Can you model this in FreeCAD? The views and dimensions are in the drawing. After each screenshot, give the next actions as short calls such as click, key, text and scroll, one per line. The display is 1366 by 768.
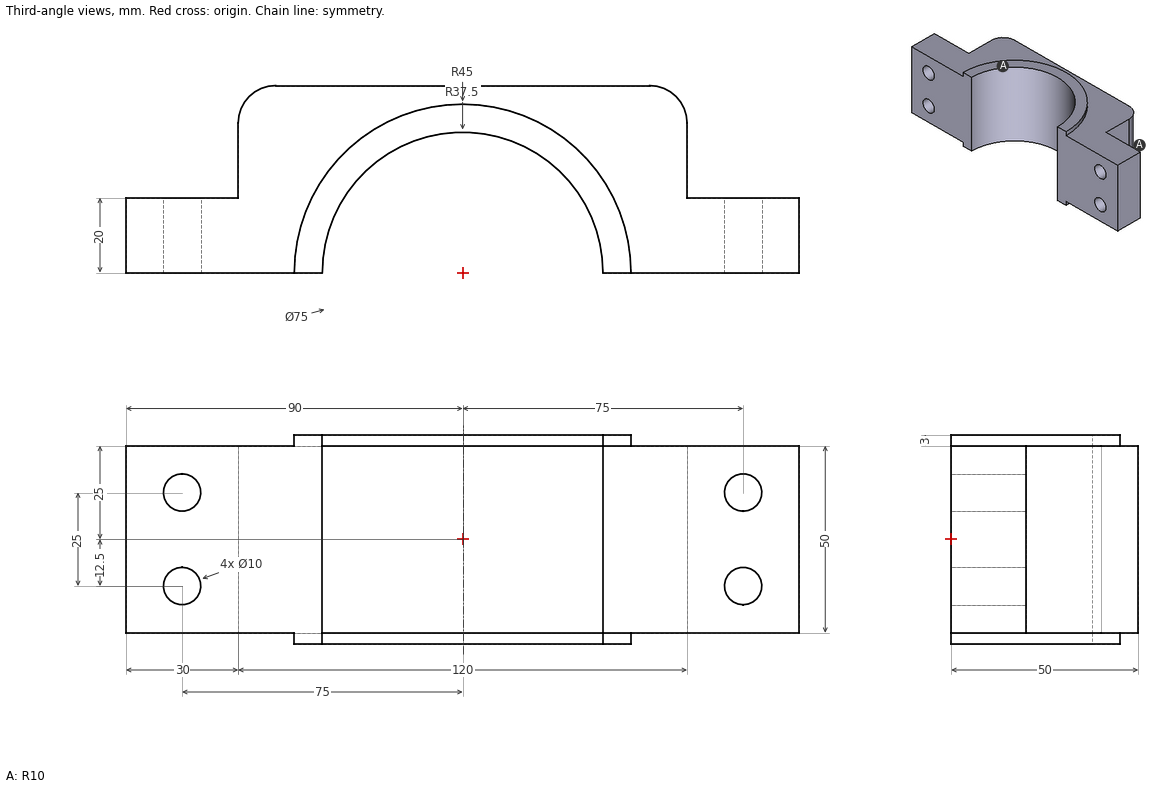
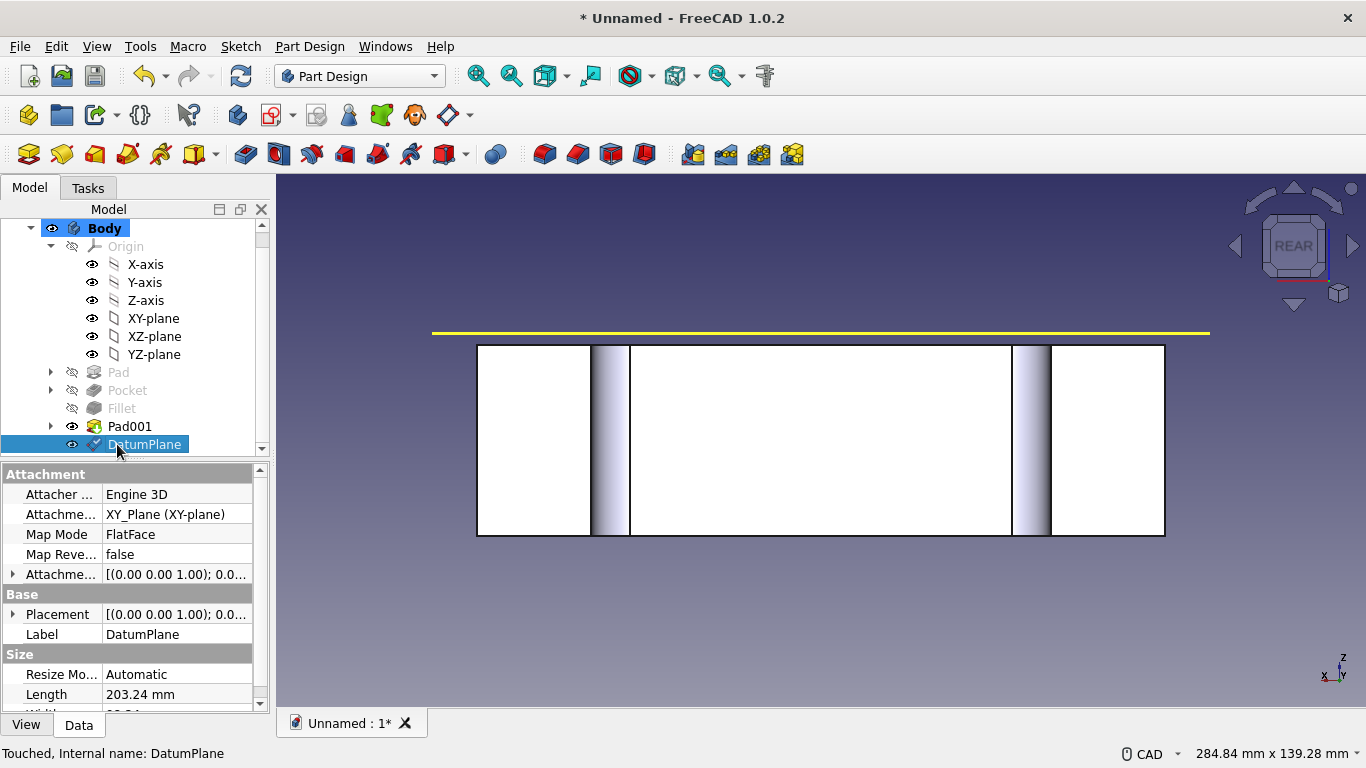
click(270, 116)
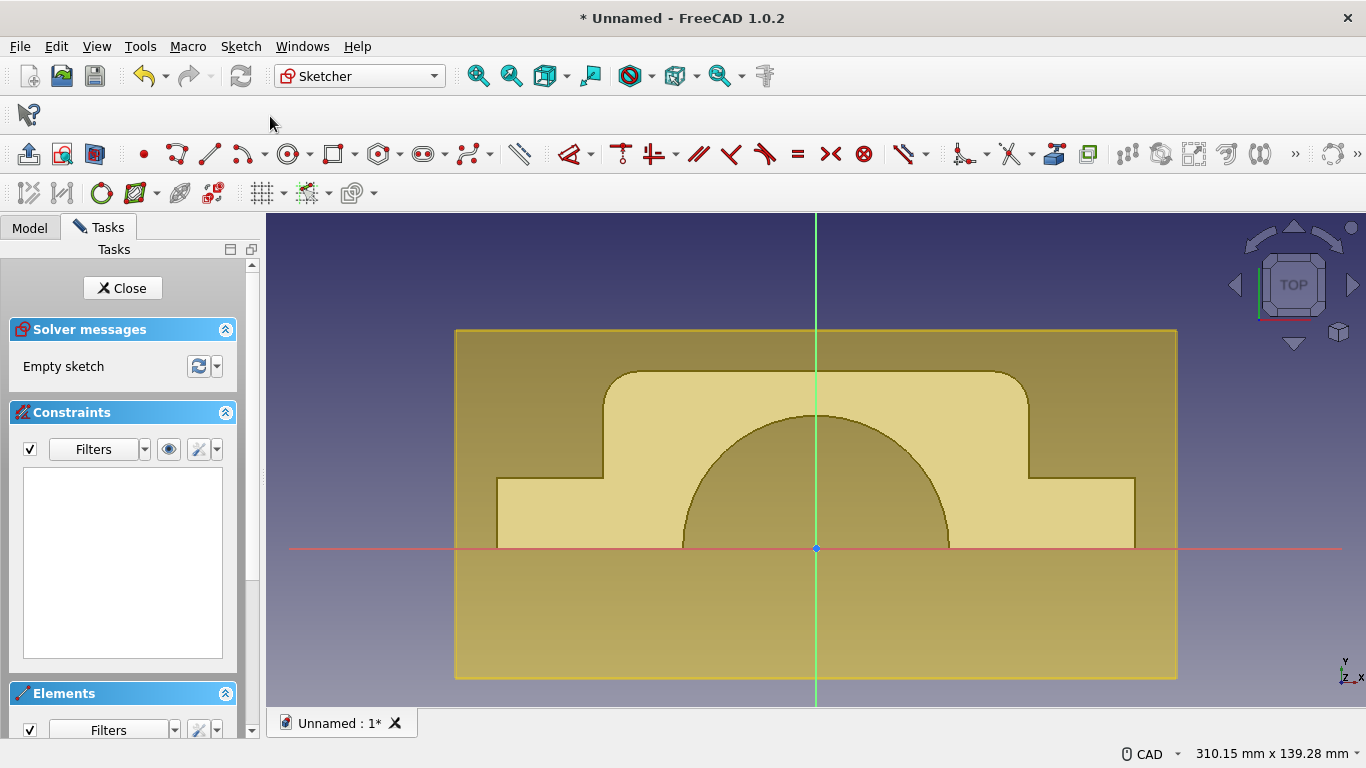
scroll(899, 480, up, 3)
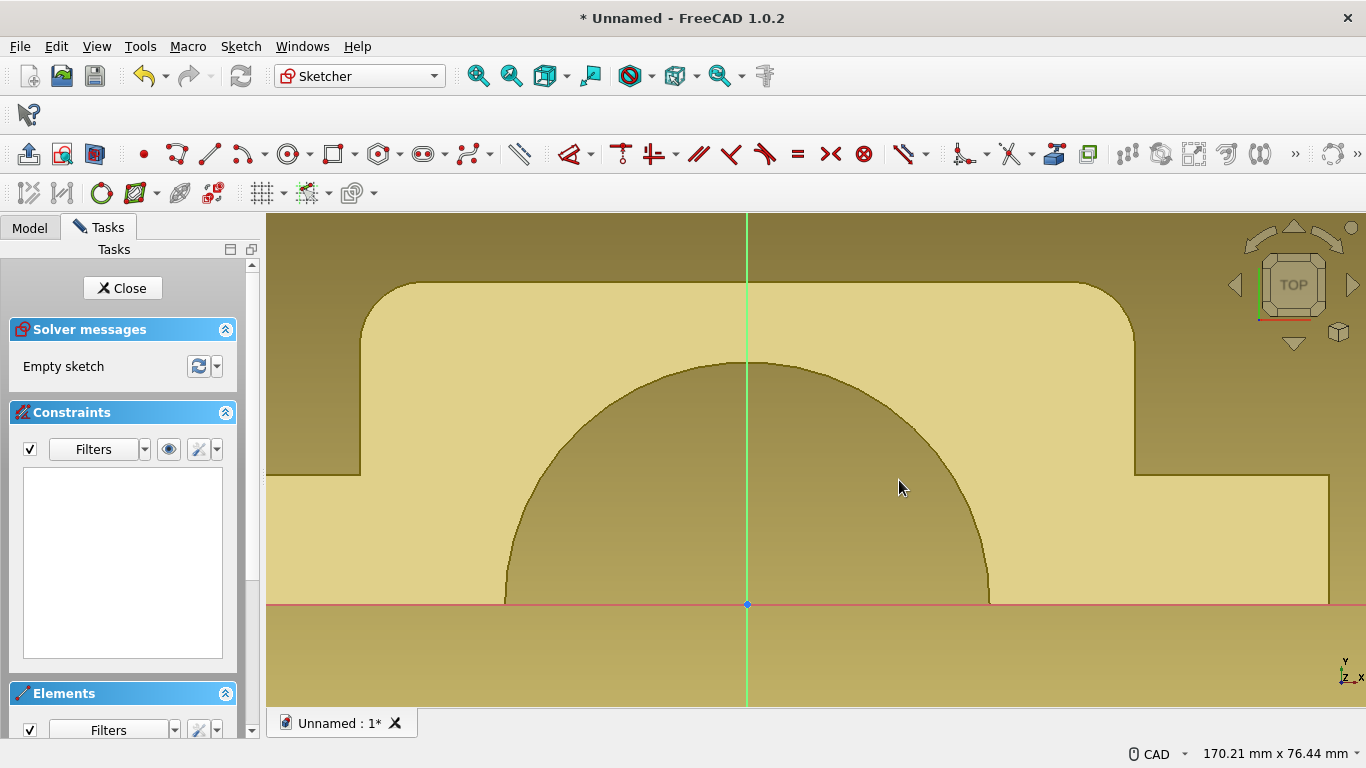
key(g)
key(l)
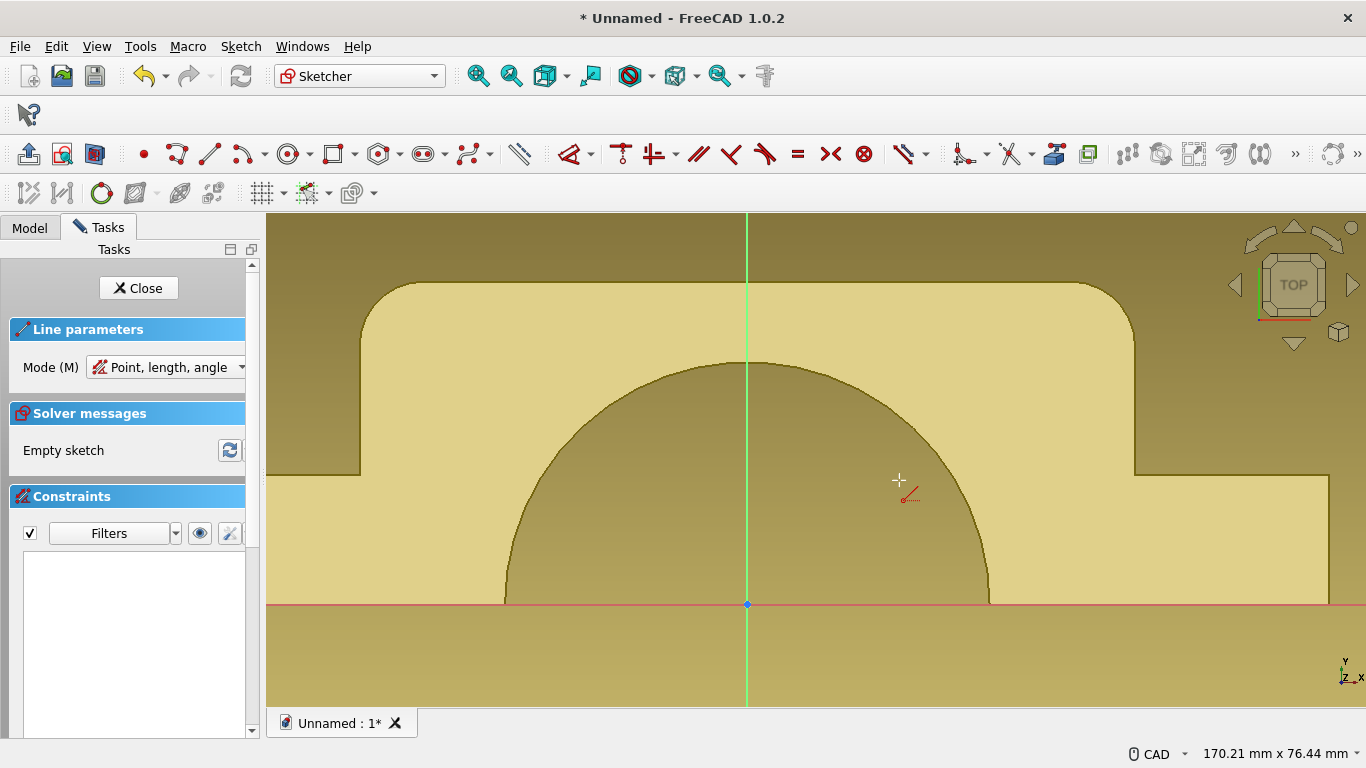
click(456, 605)
click(505, 596)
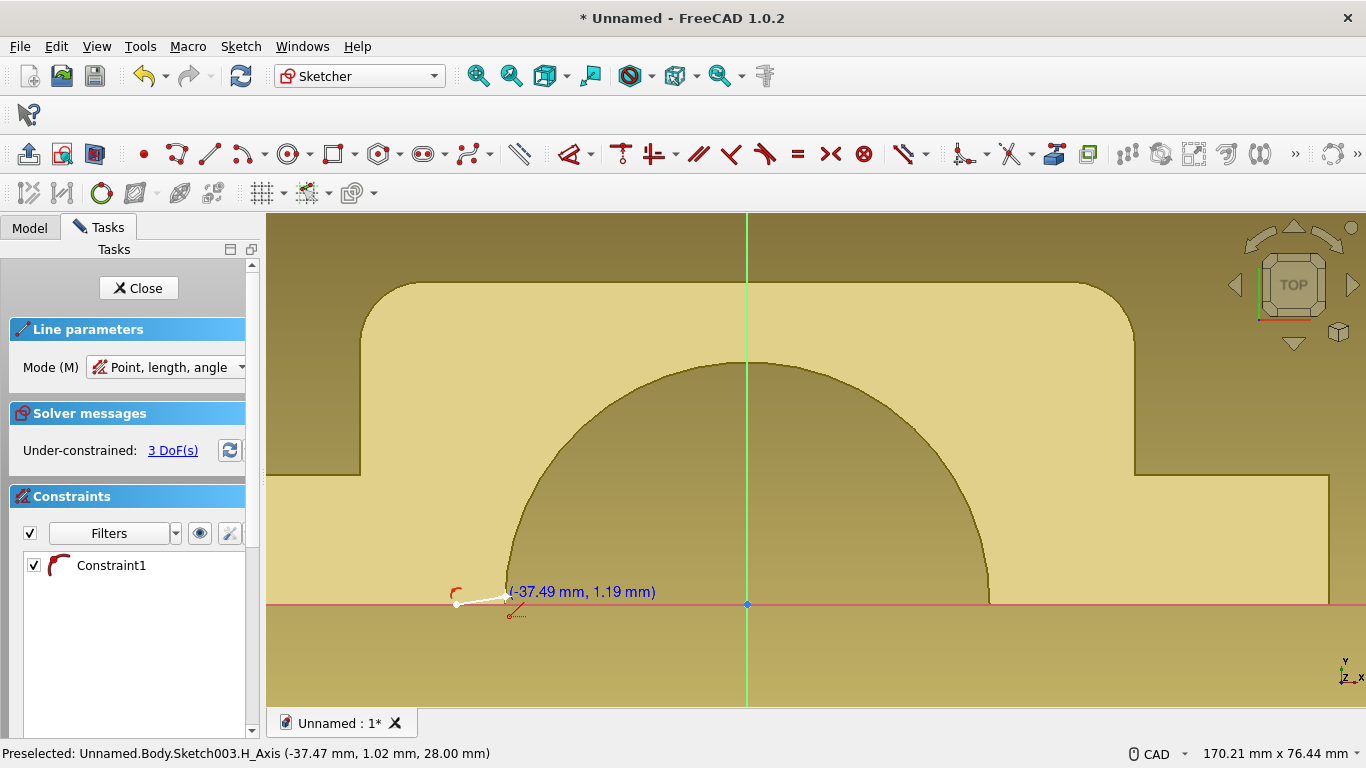
click(990, 605)
click(1038, 596)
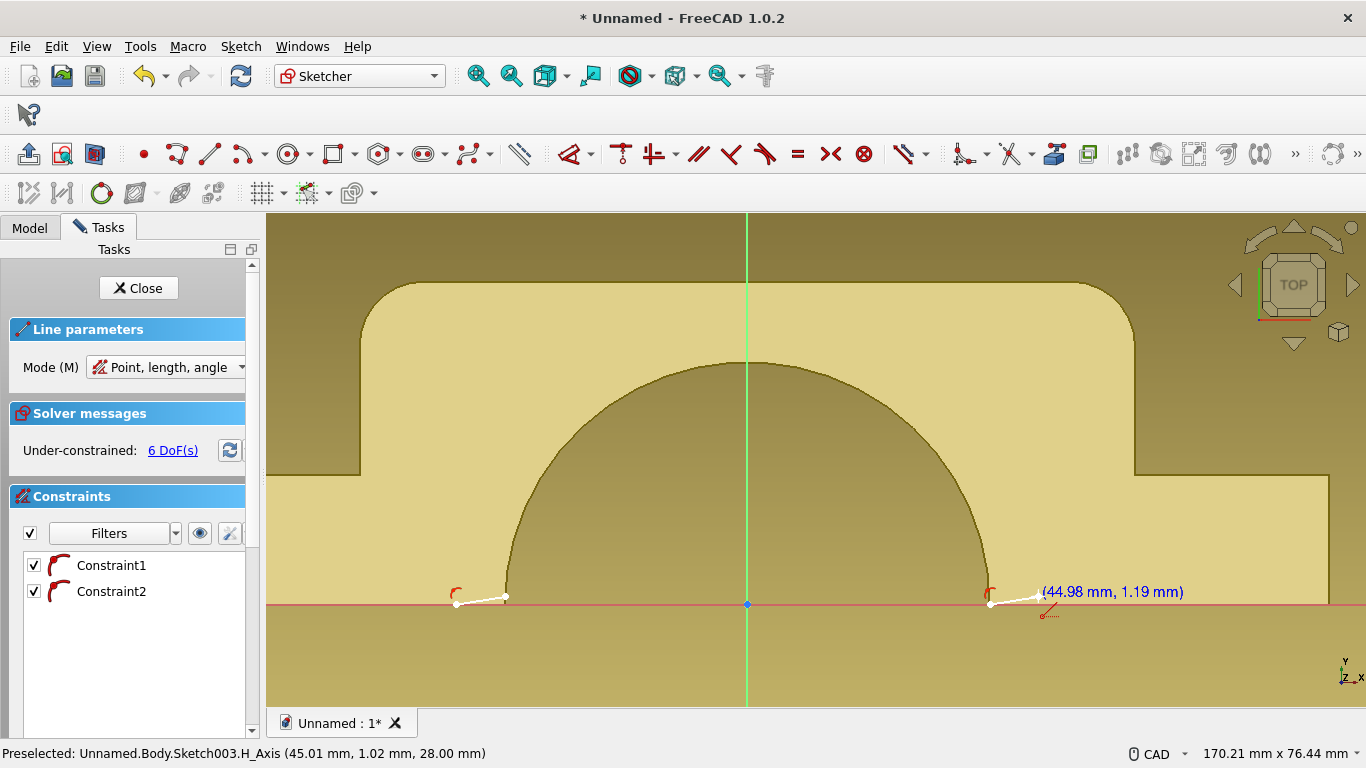
key(g)
key(3)
key(a)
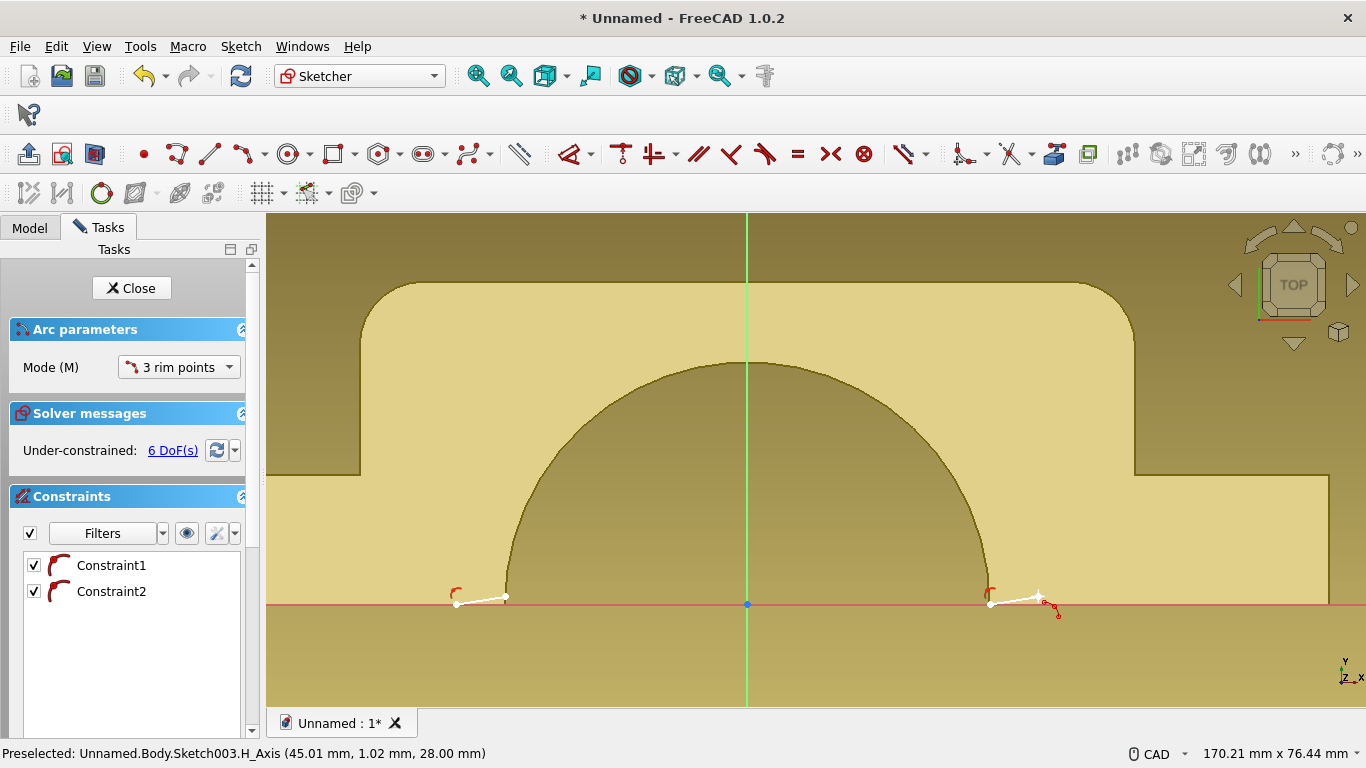
click(505, 597)
click(990, 605)
click(822, 374)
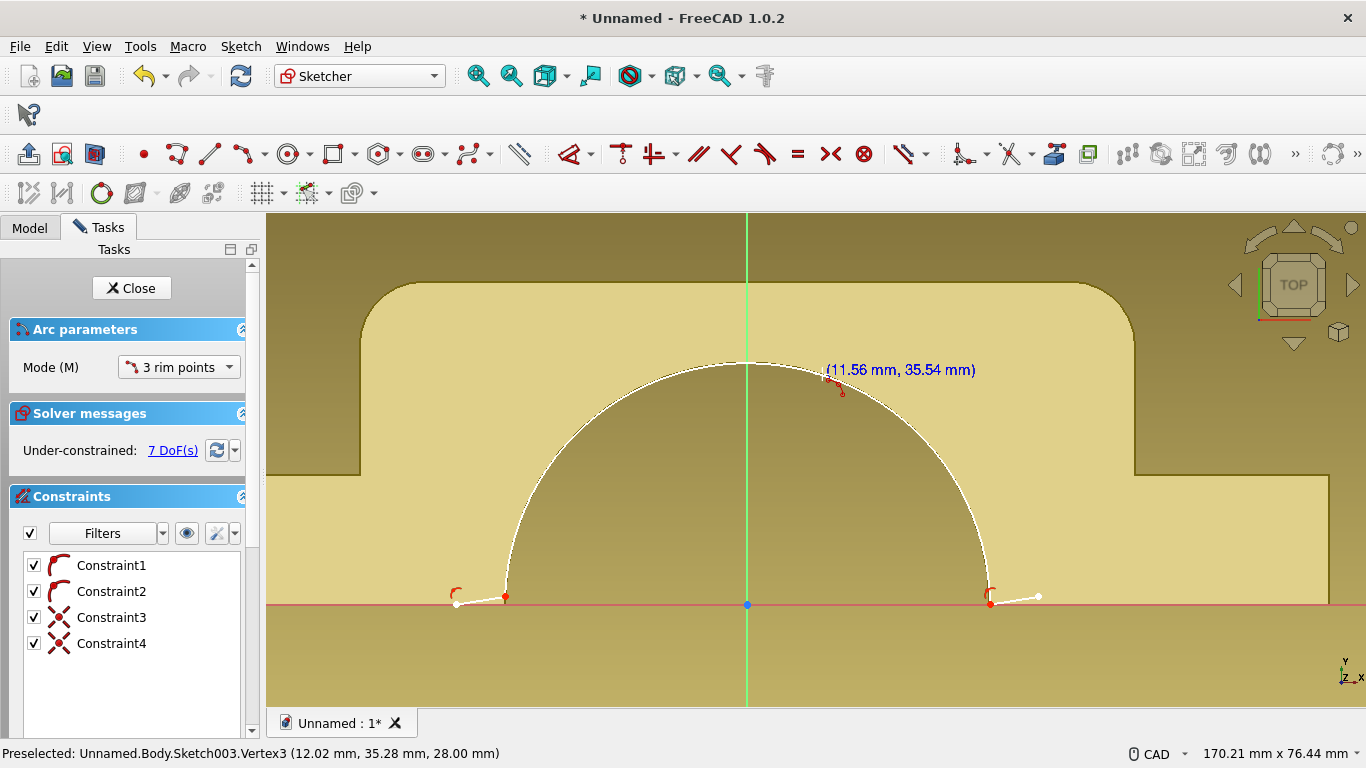
click(1038, 597)
click(456, 605)
click(837, 328)
key(Escape)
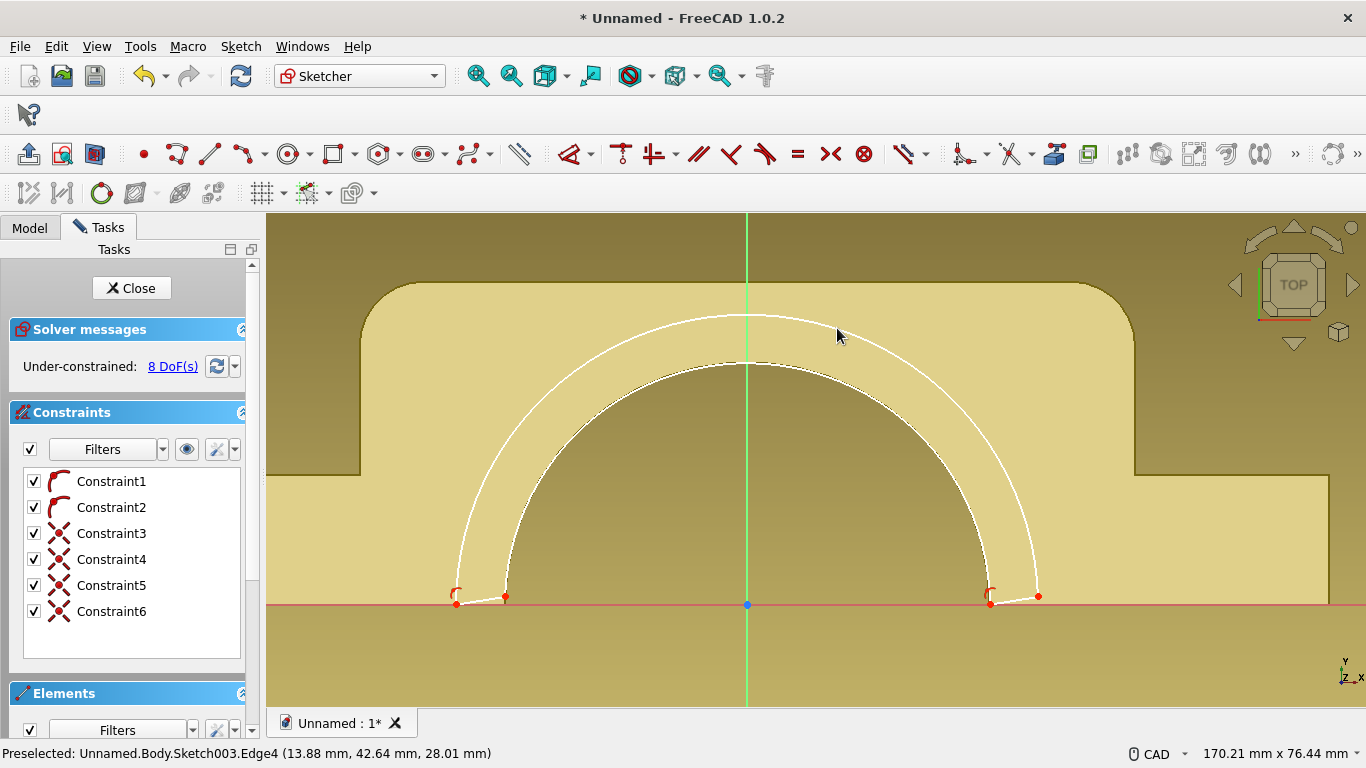
click(471, 602)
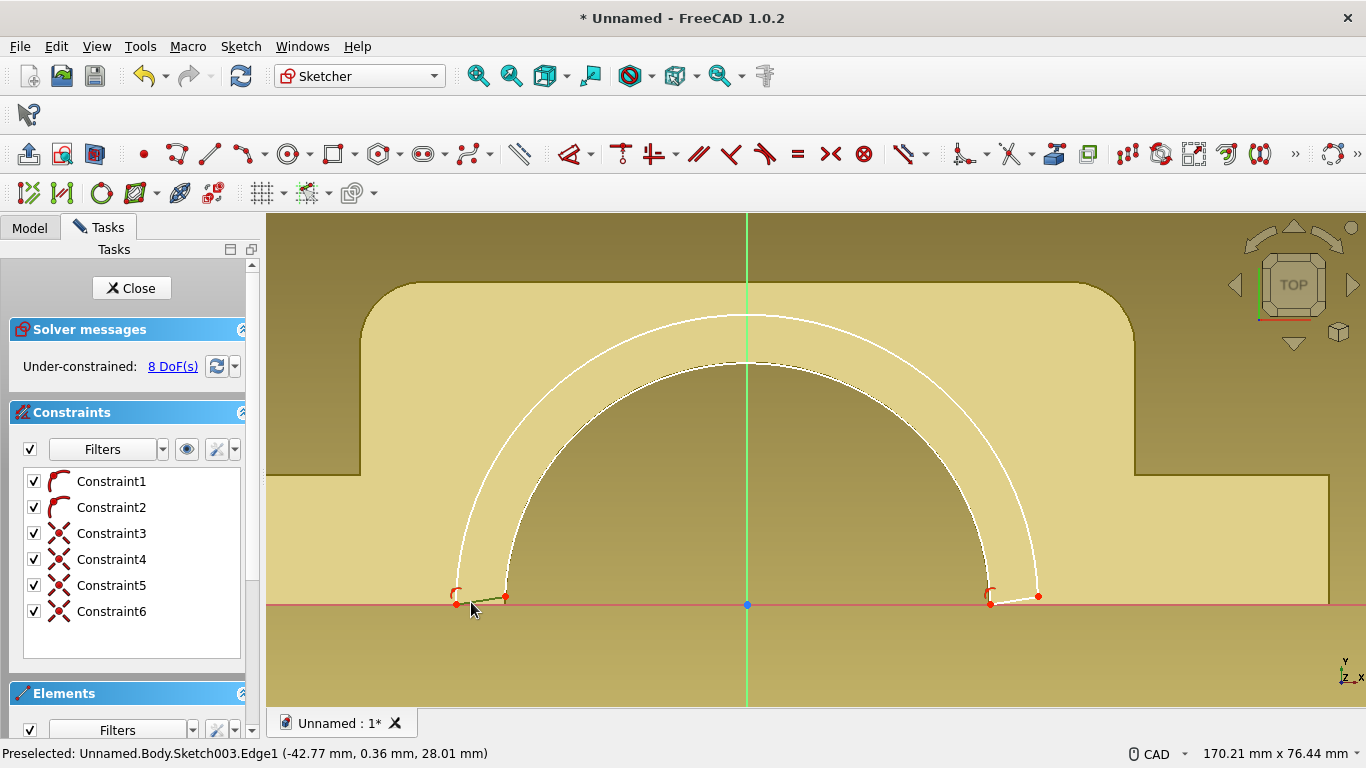
key(h)